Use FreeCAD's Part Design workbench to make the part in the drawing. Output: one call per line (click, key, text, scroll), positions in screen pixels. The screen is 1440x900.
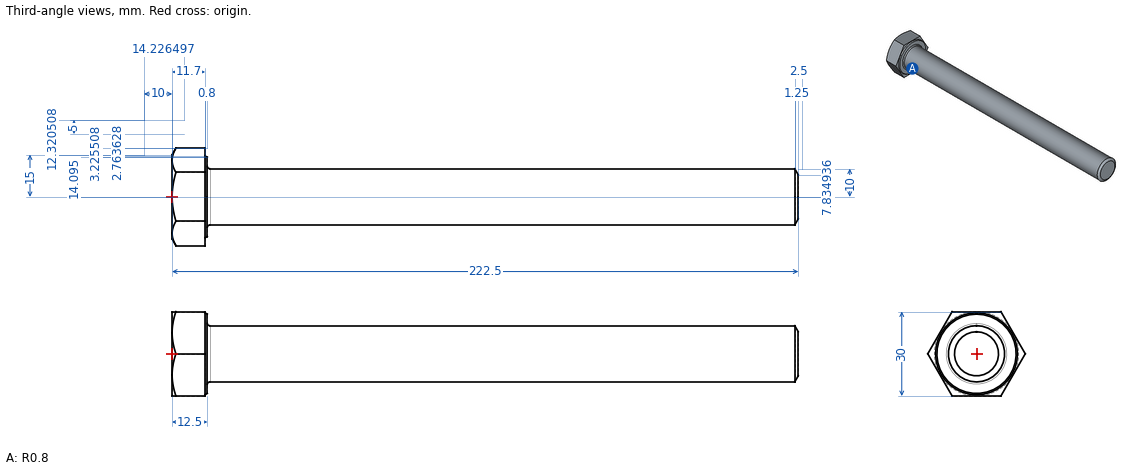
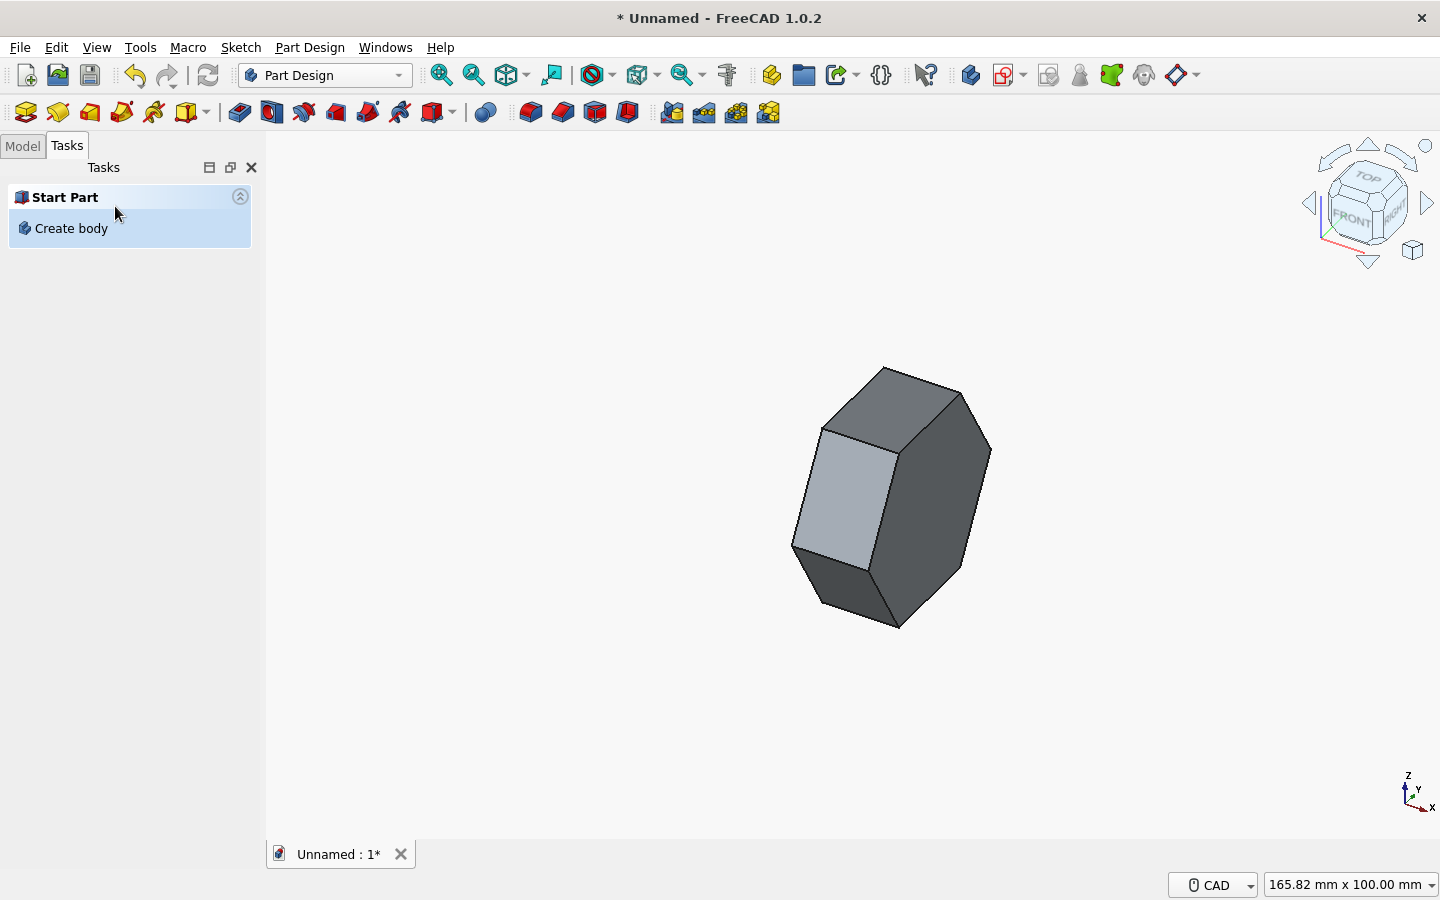
click(1004, 76)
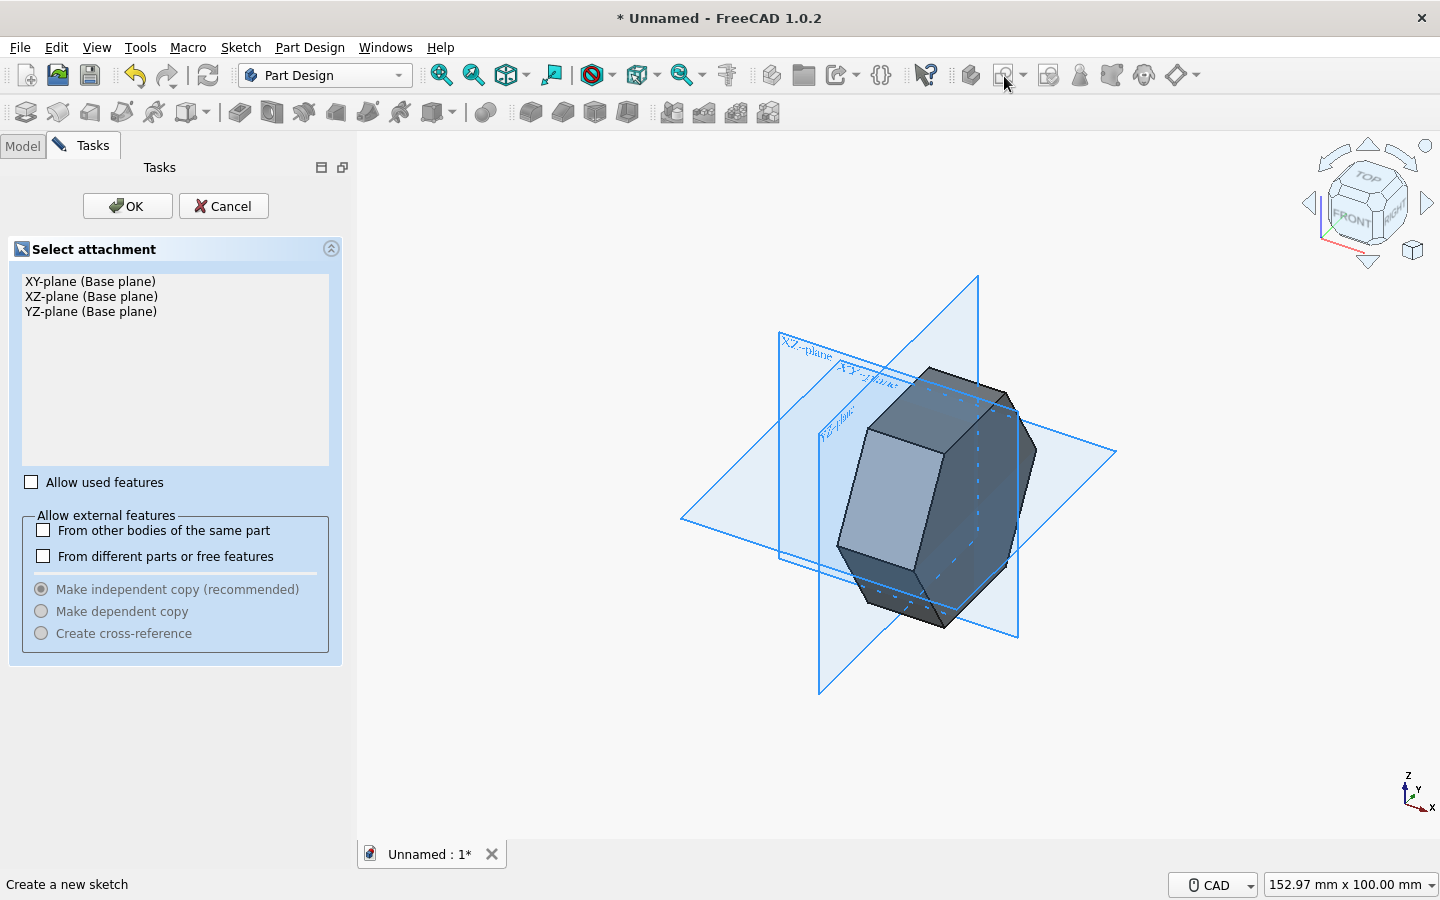
click(82, 282)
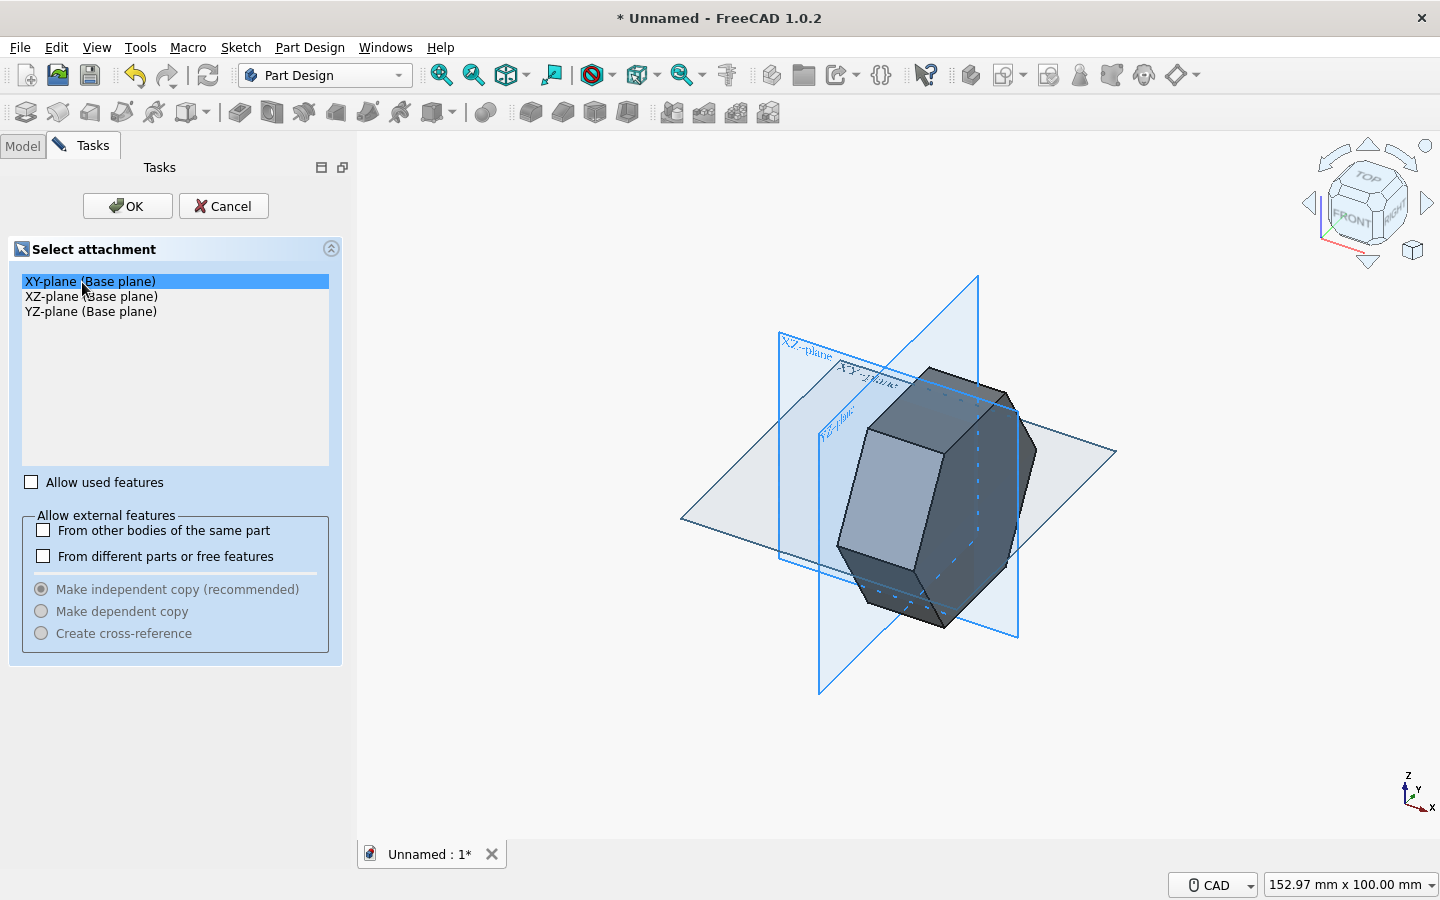
click(128, 206)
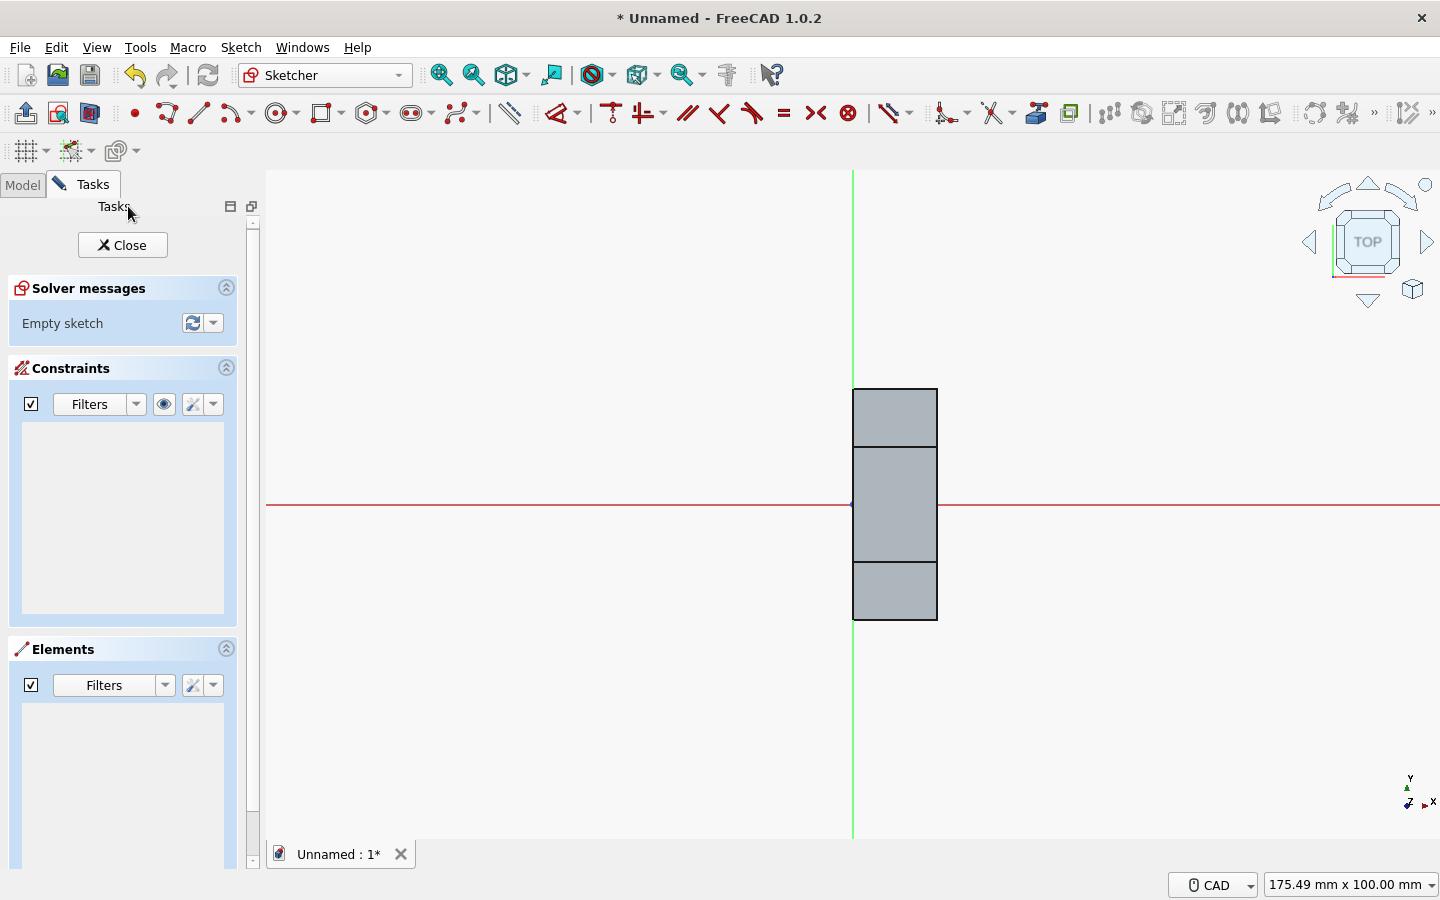
click(90, 114)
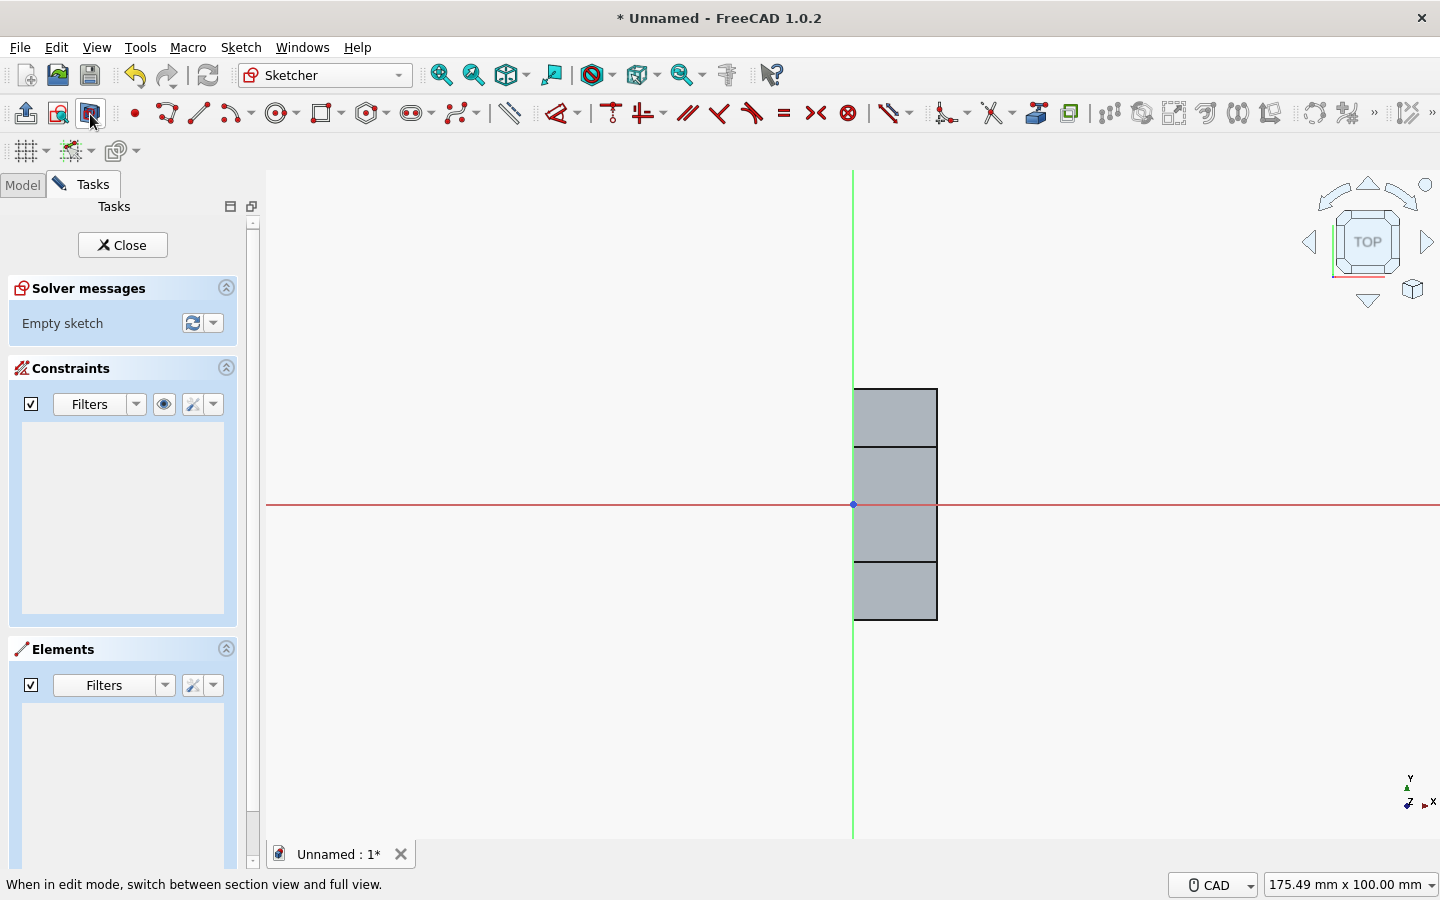
scroll(294, 532, down, 4)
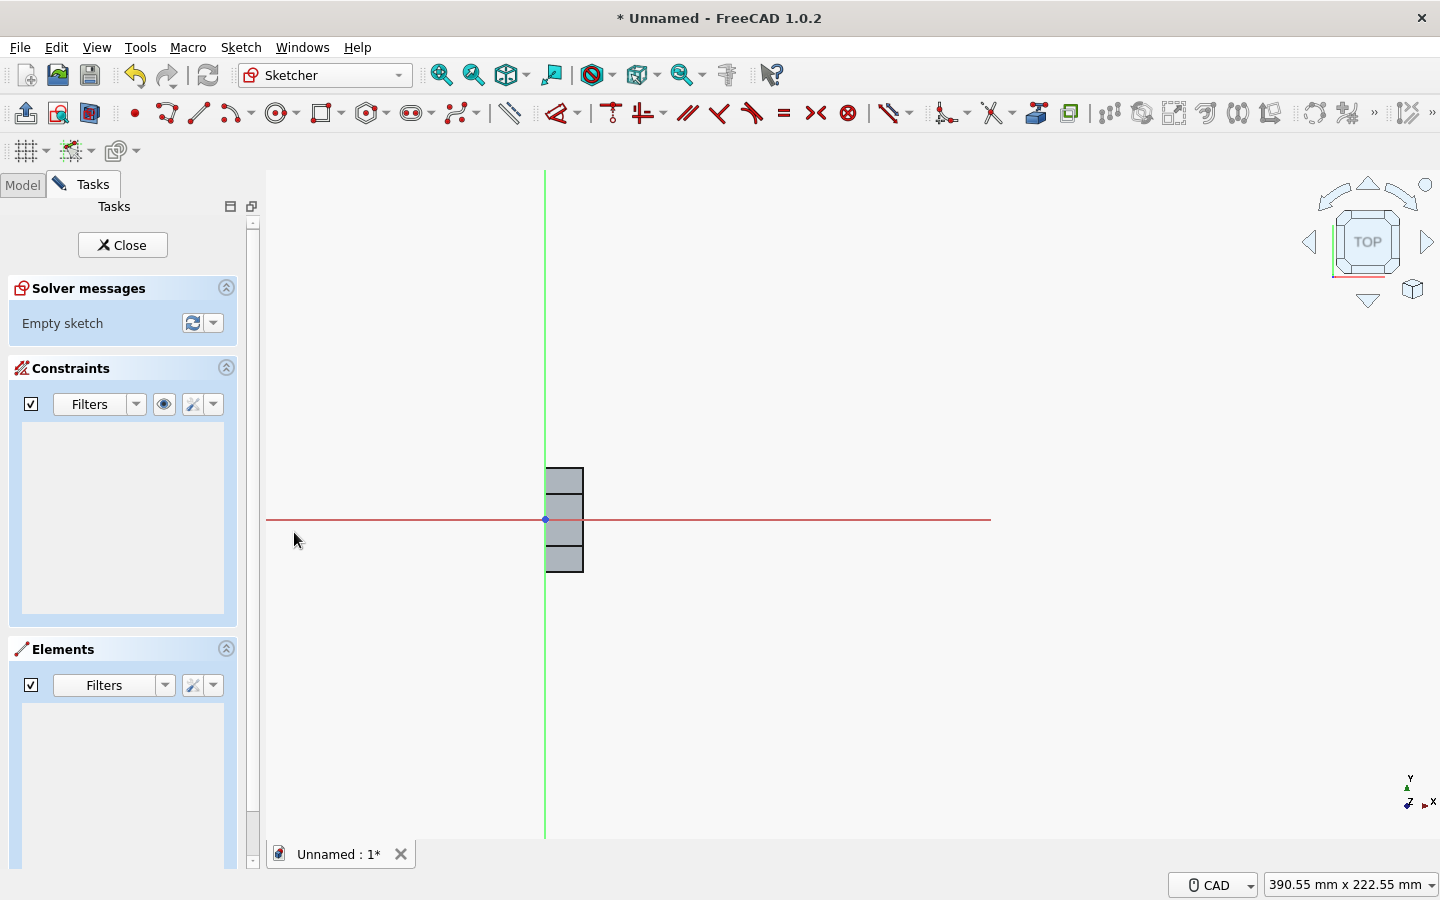
click(322, 114)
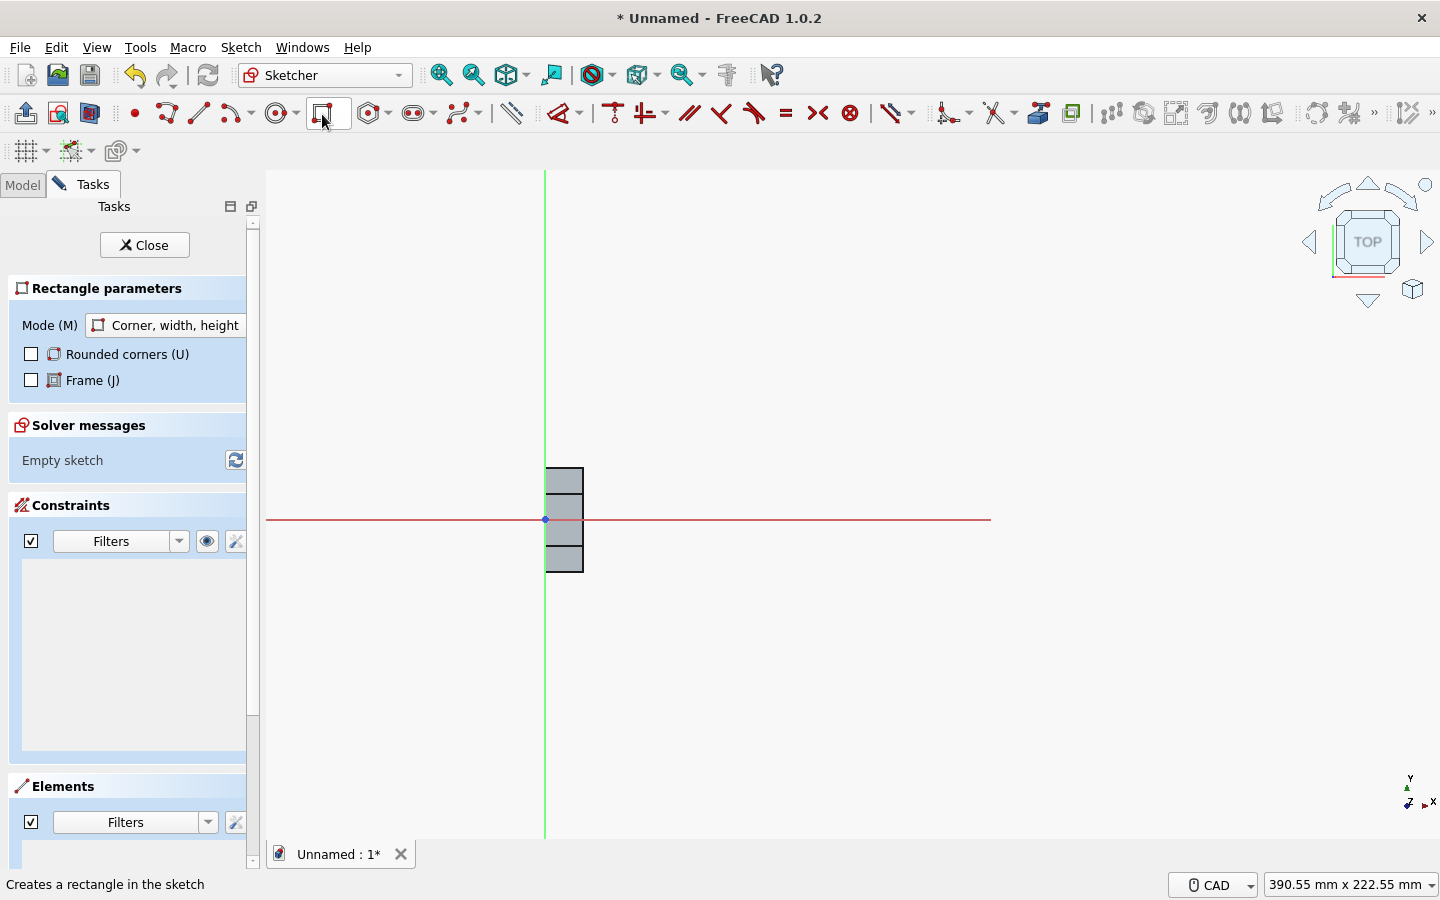
click(545, 520)
move(1214, 490)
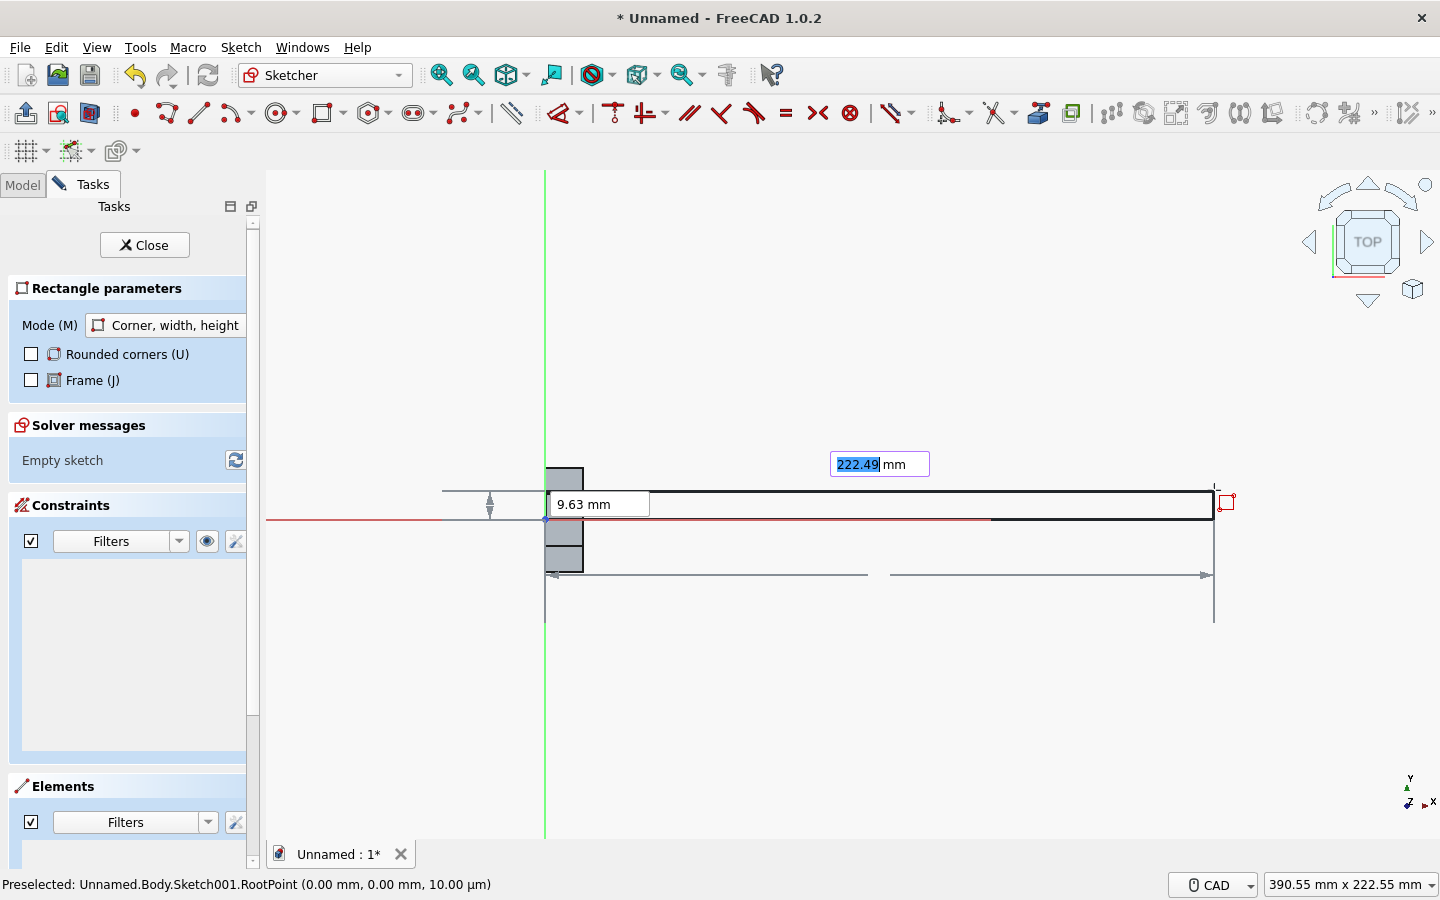
text(222.5)
key(Tab)
text(10)
key(Return)
key(Escape)